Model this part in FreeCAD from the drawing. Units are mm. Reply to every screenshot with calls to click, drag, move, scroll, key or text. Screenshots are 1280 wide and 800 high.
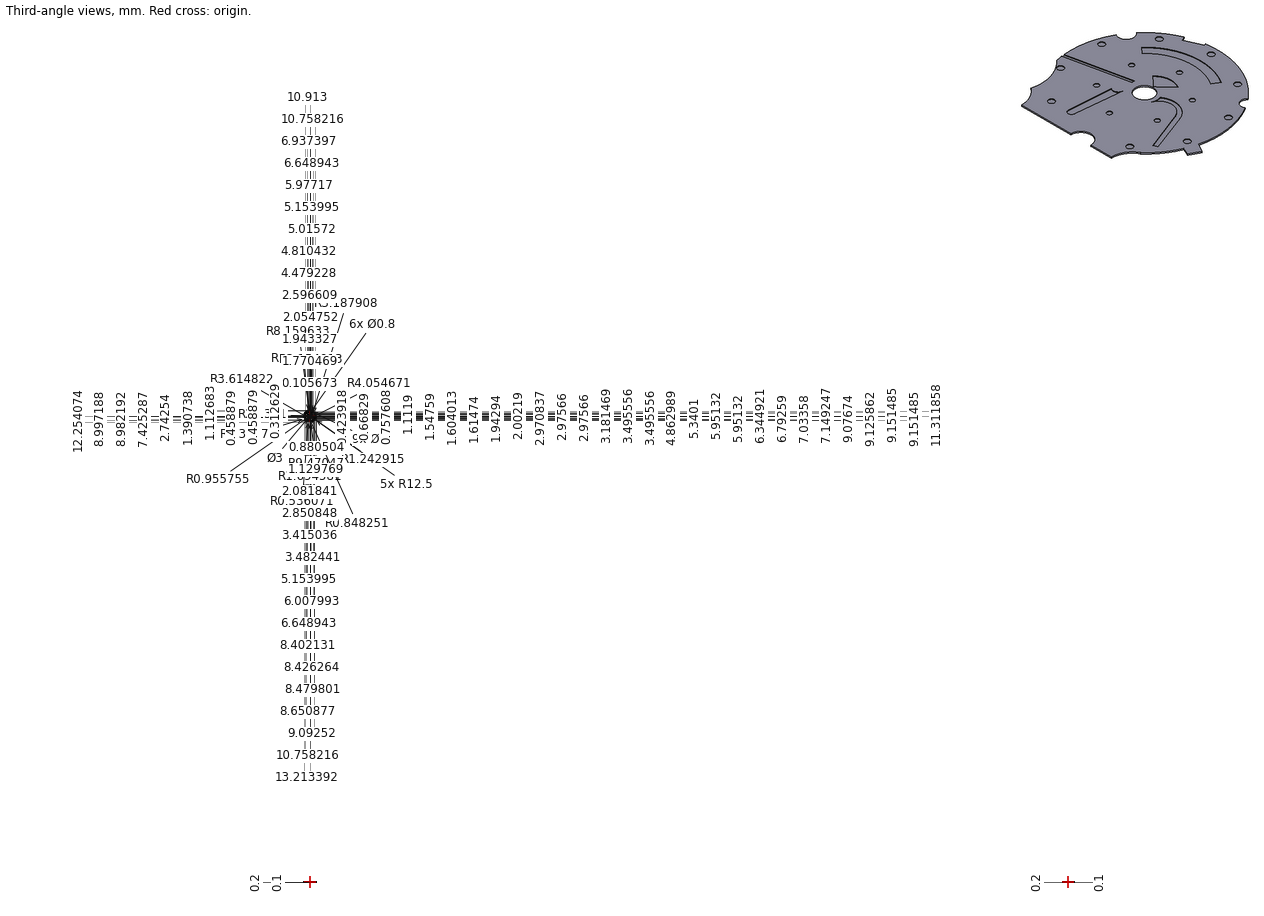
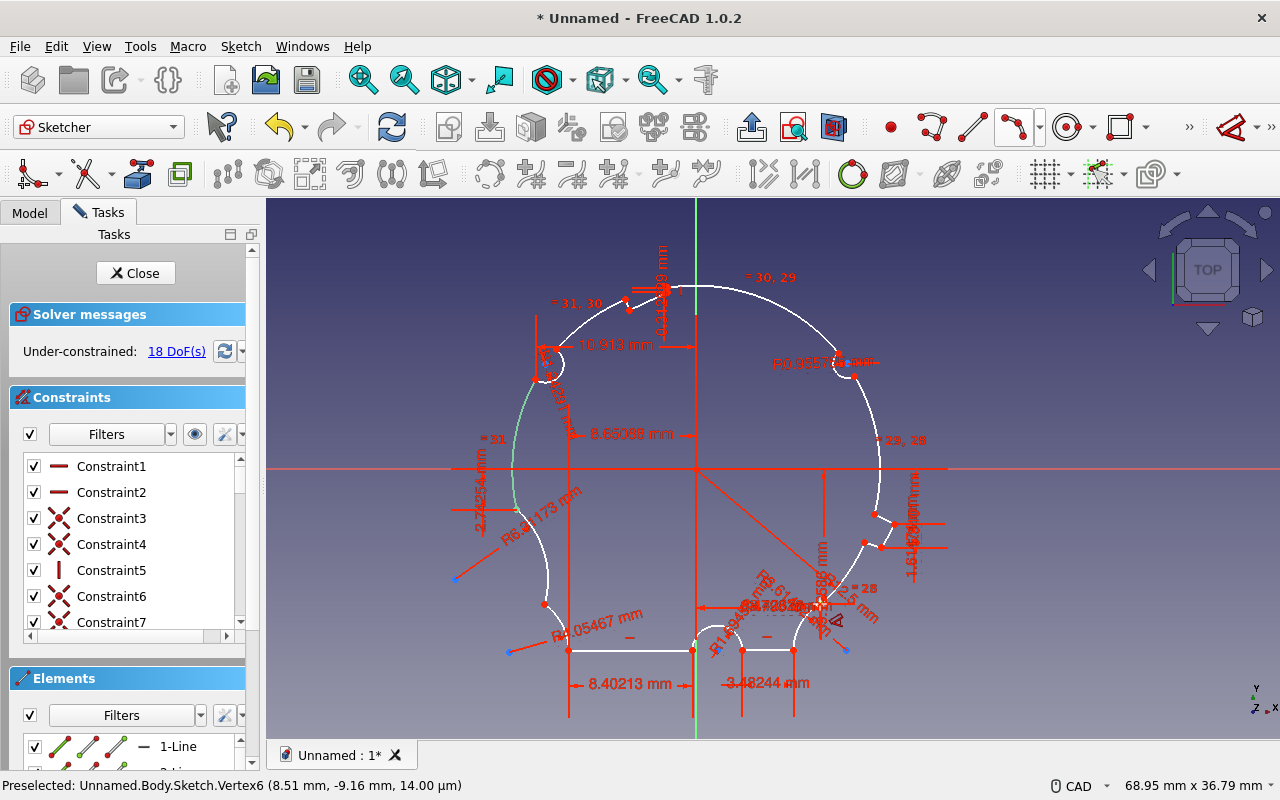
click(865, 543)
click(899, 489)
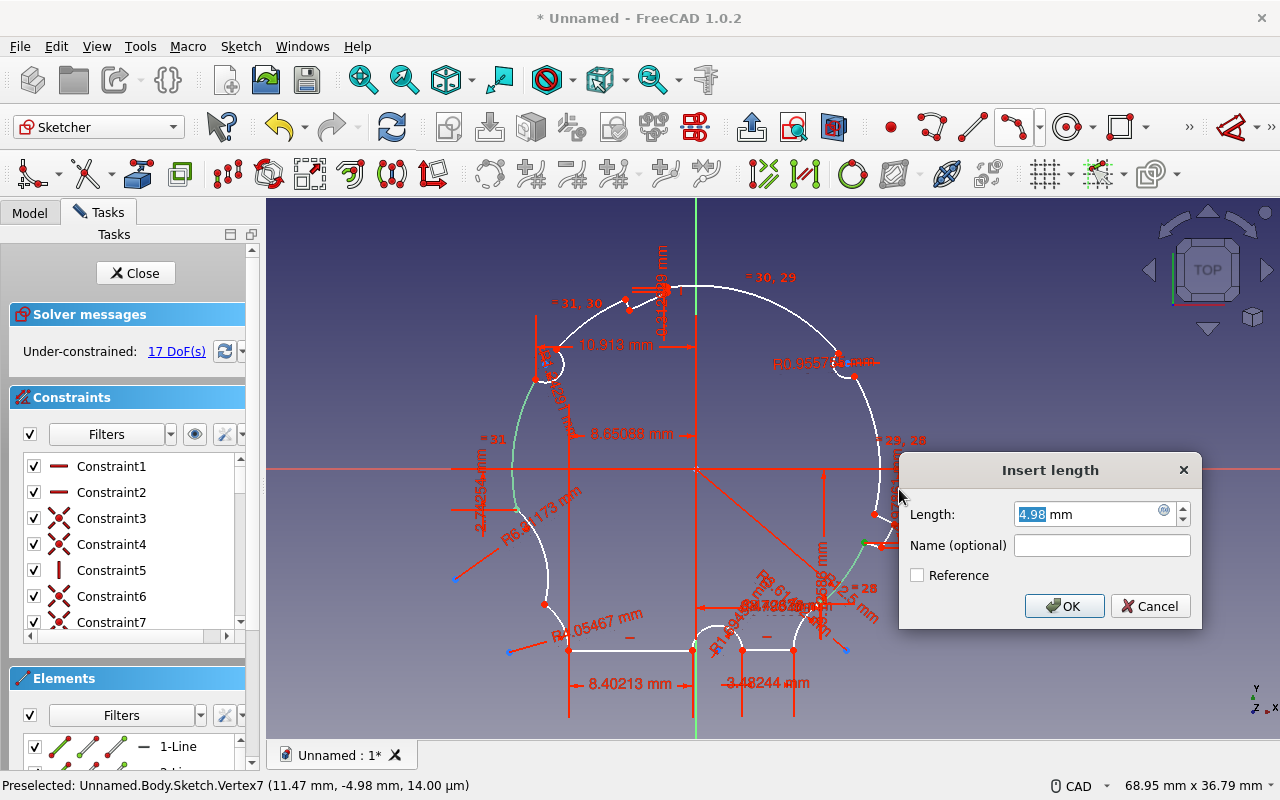
text(4.862989)
key(Return)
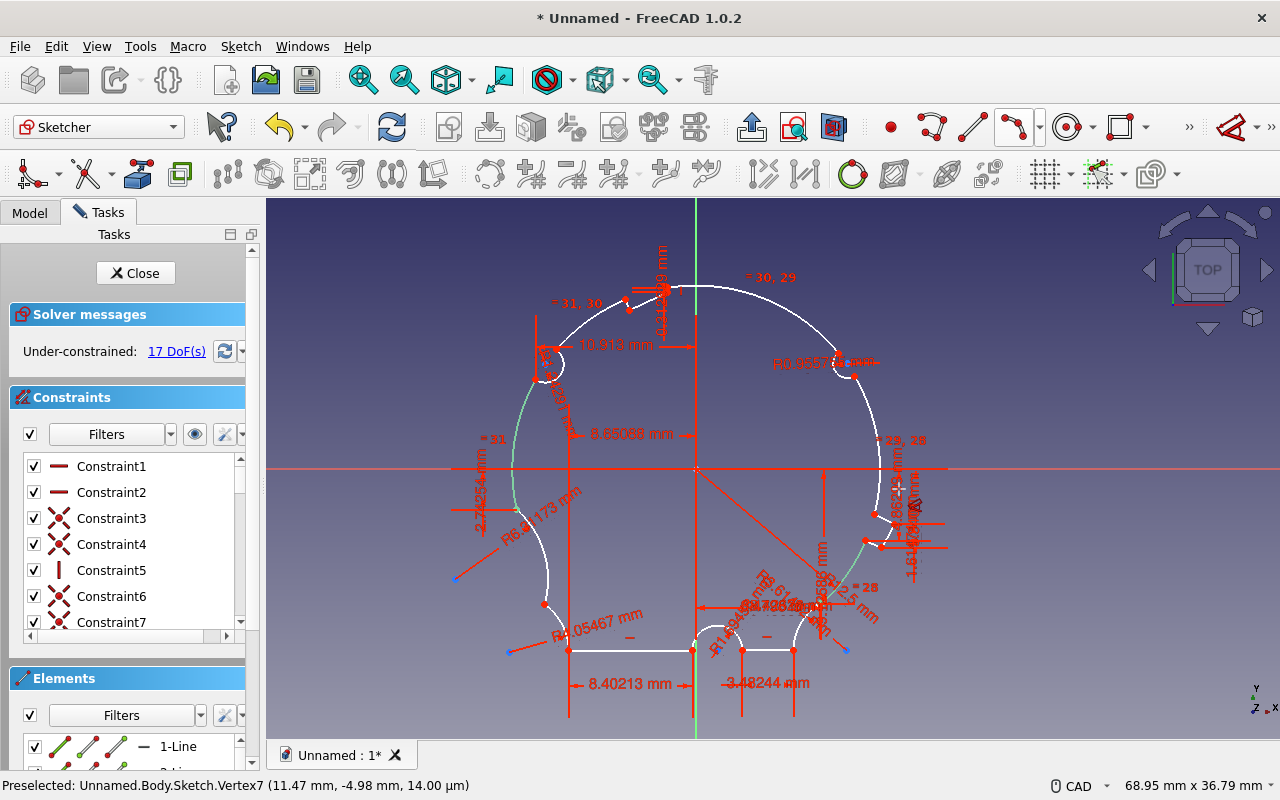
click(874, 514)
click(662, 492)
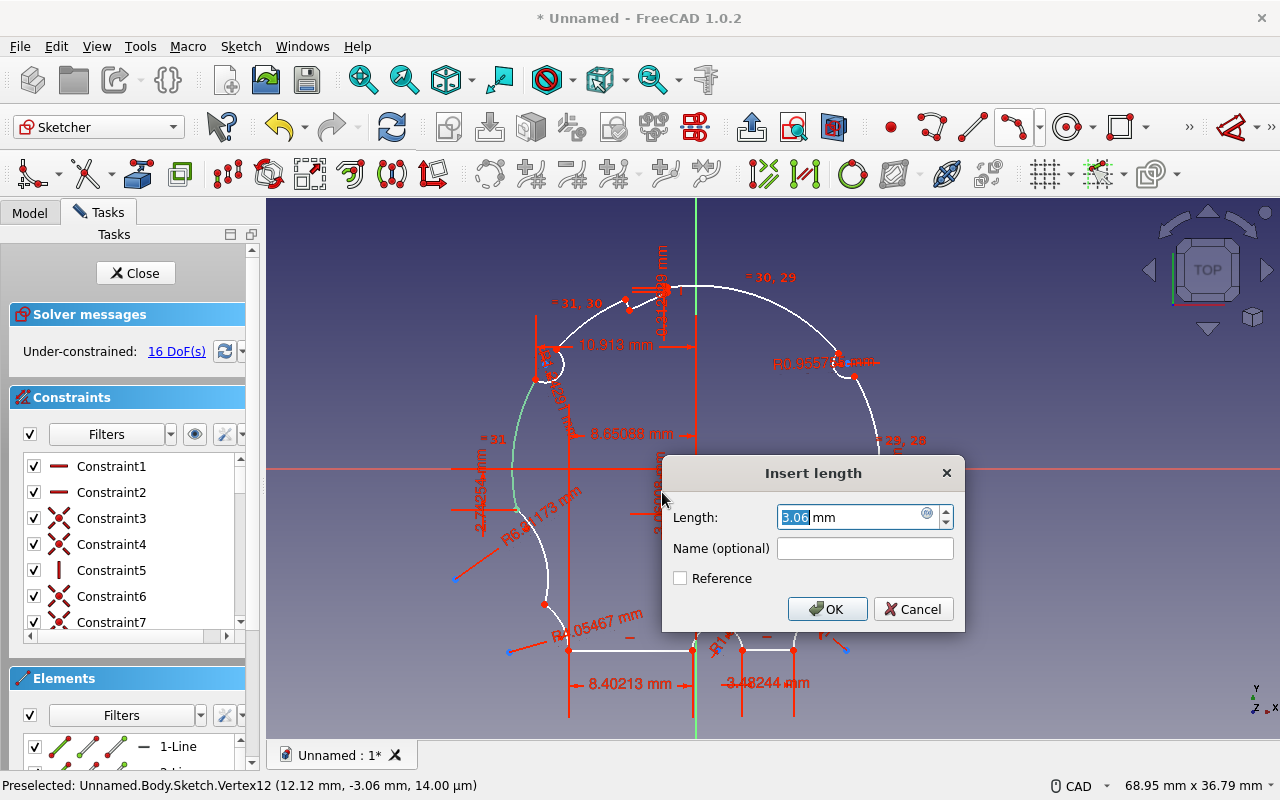
text(2.970837)
key(Return)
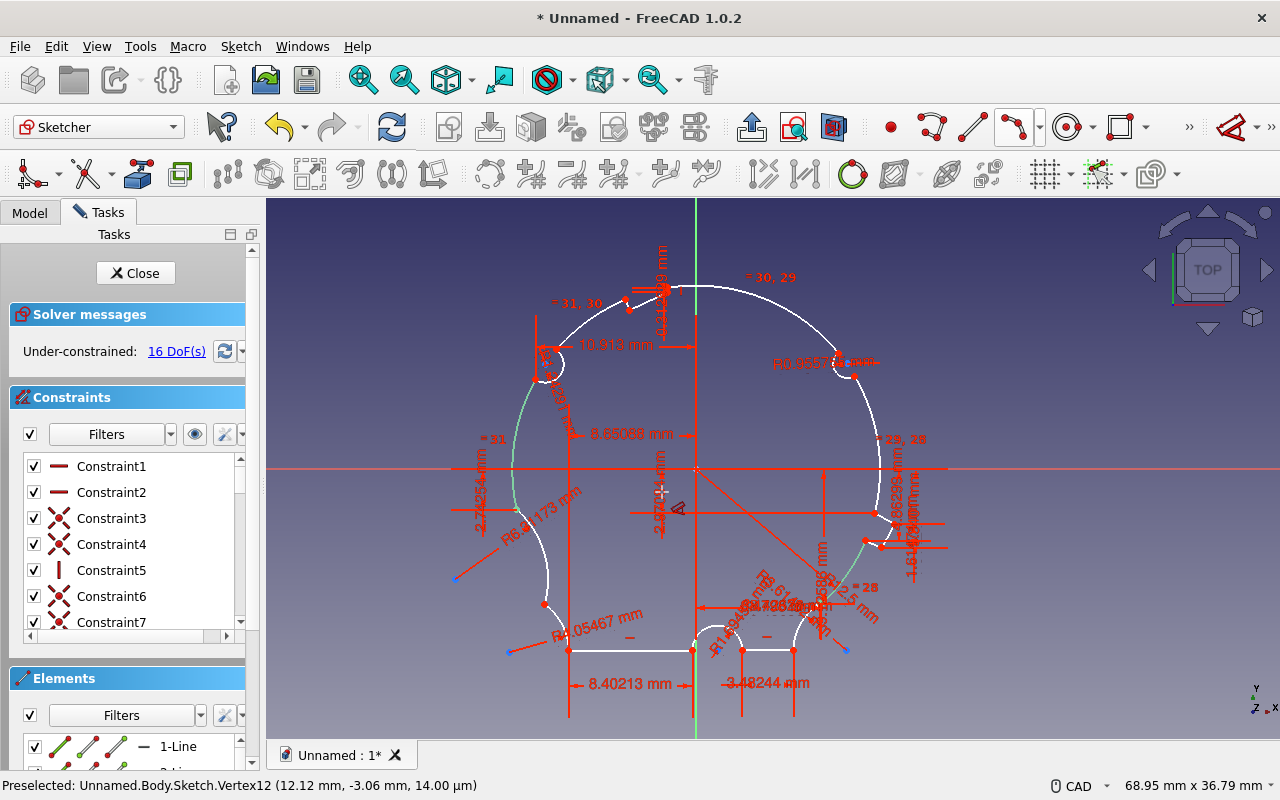
scroll(668, 288, up, 5)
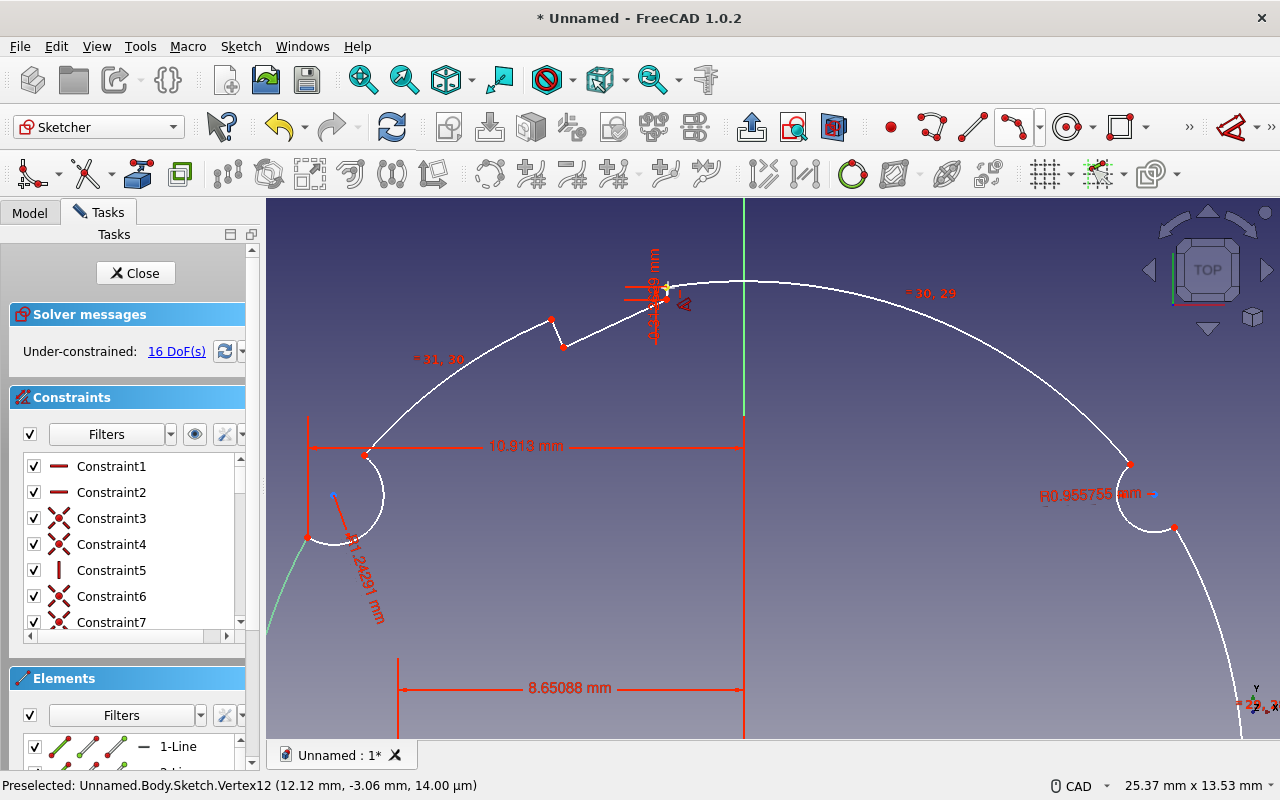
click(667, 287)
click(705, 253)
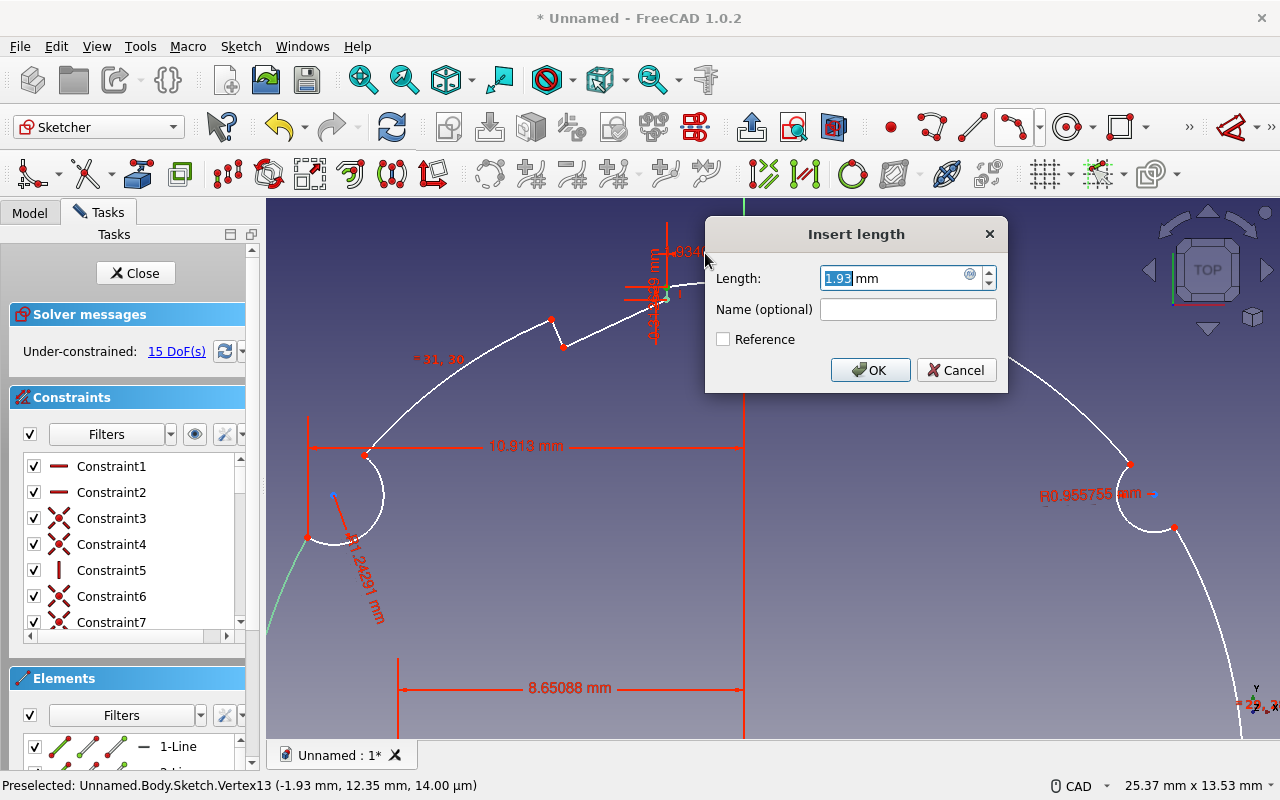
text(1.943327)
key(Return)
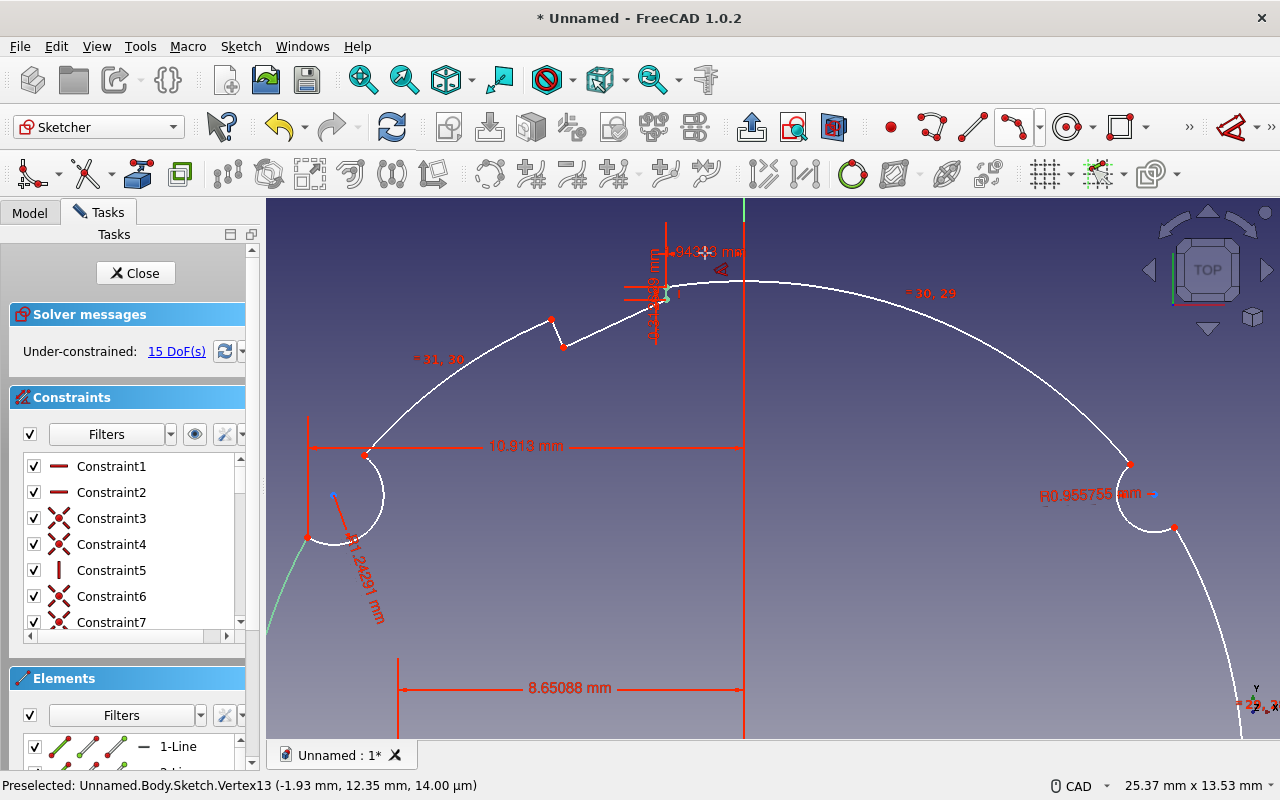
click(564, 348)
click(612, 266)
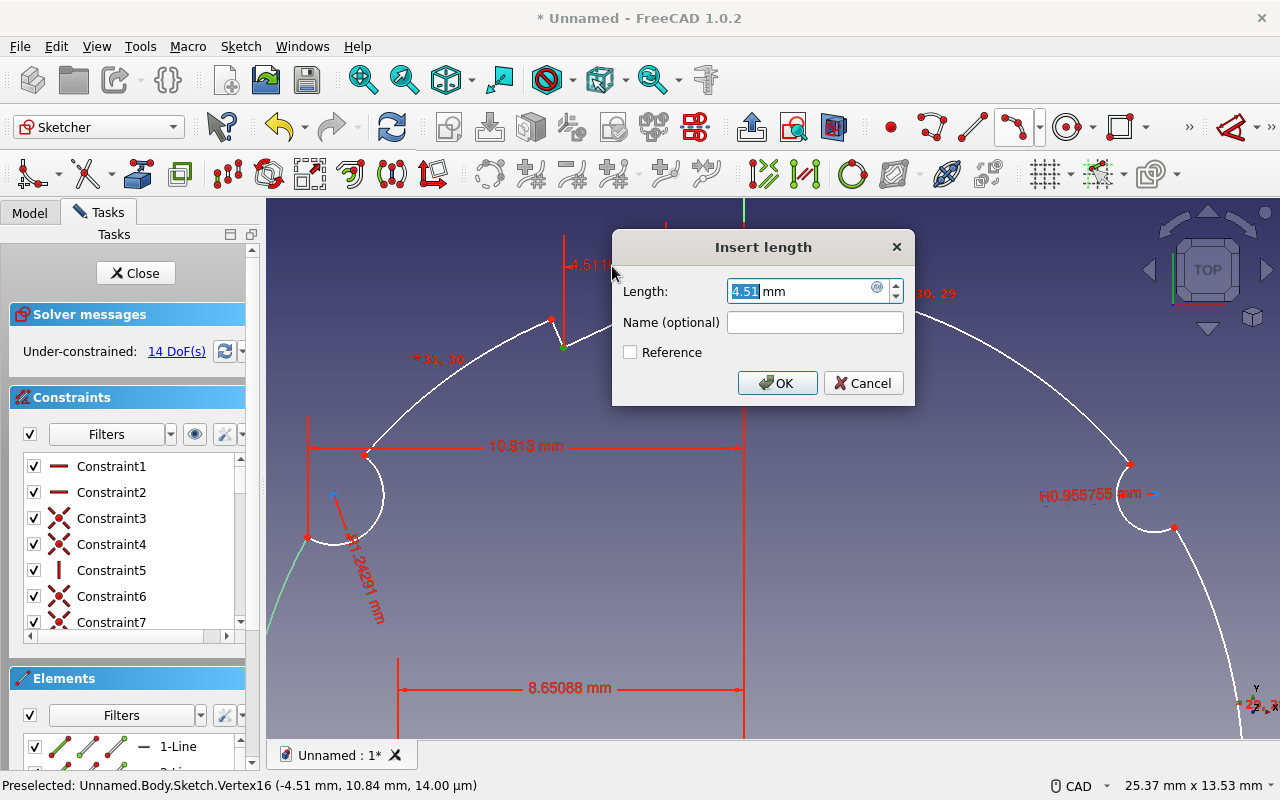
text(4.479228)
key(Return)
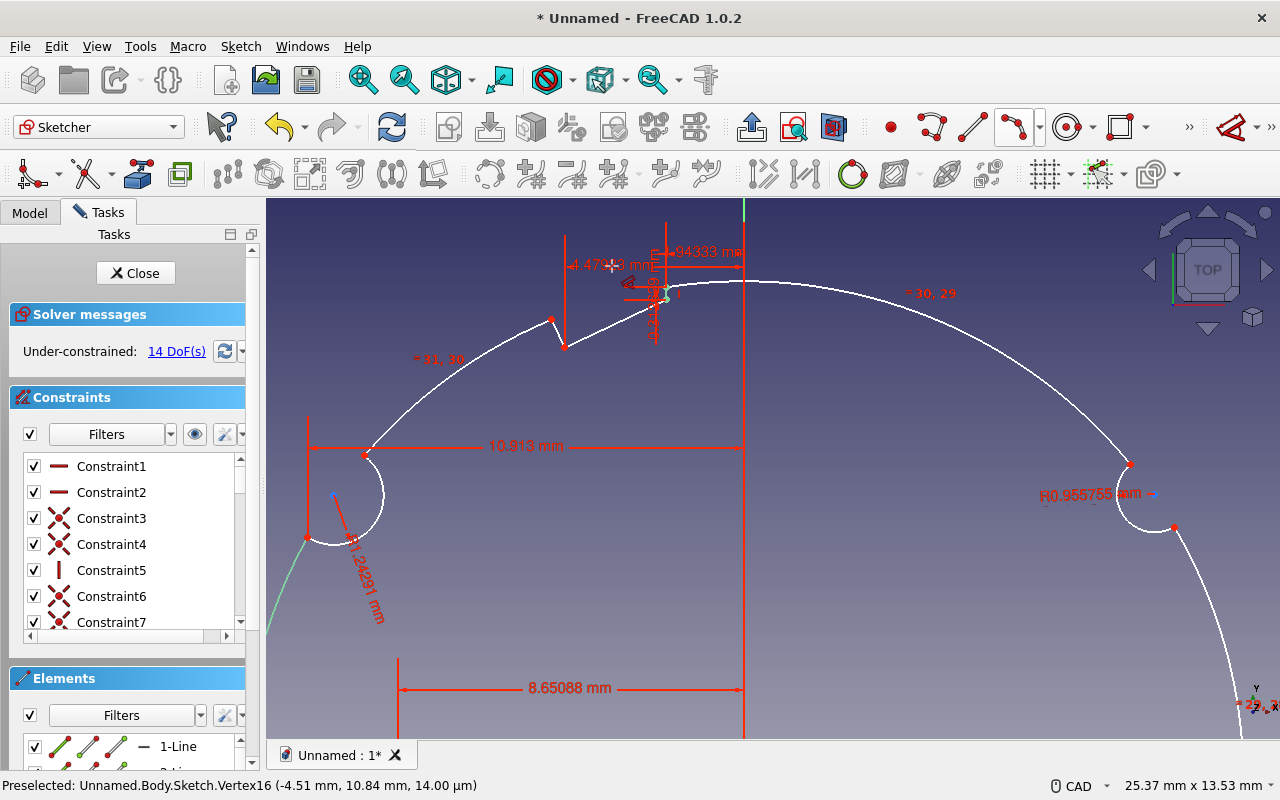
click(552, 320)
click(604, 238)